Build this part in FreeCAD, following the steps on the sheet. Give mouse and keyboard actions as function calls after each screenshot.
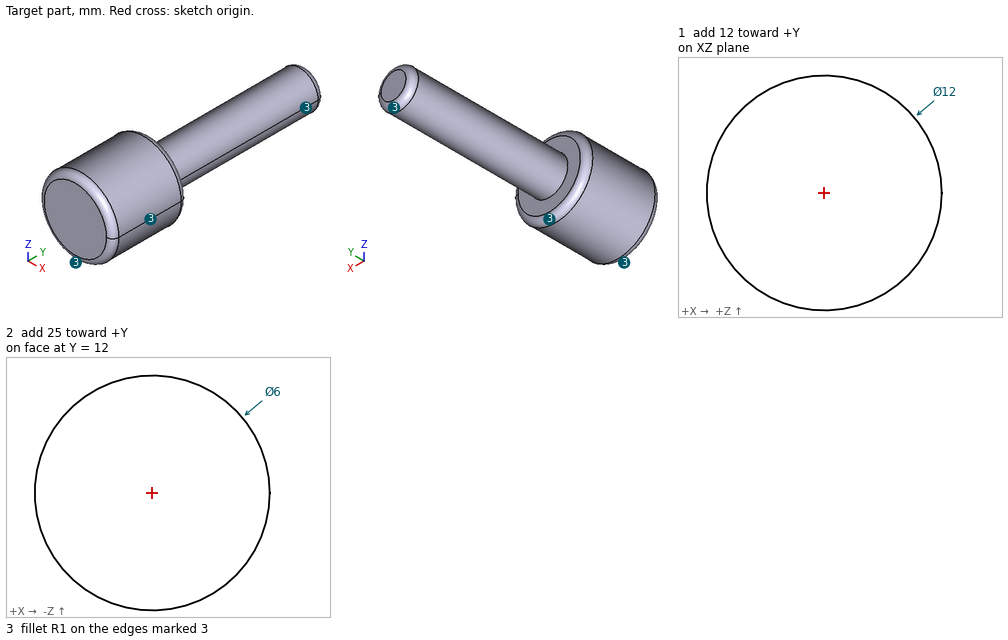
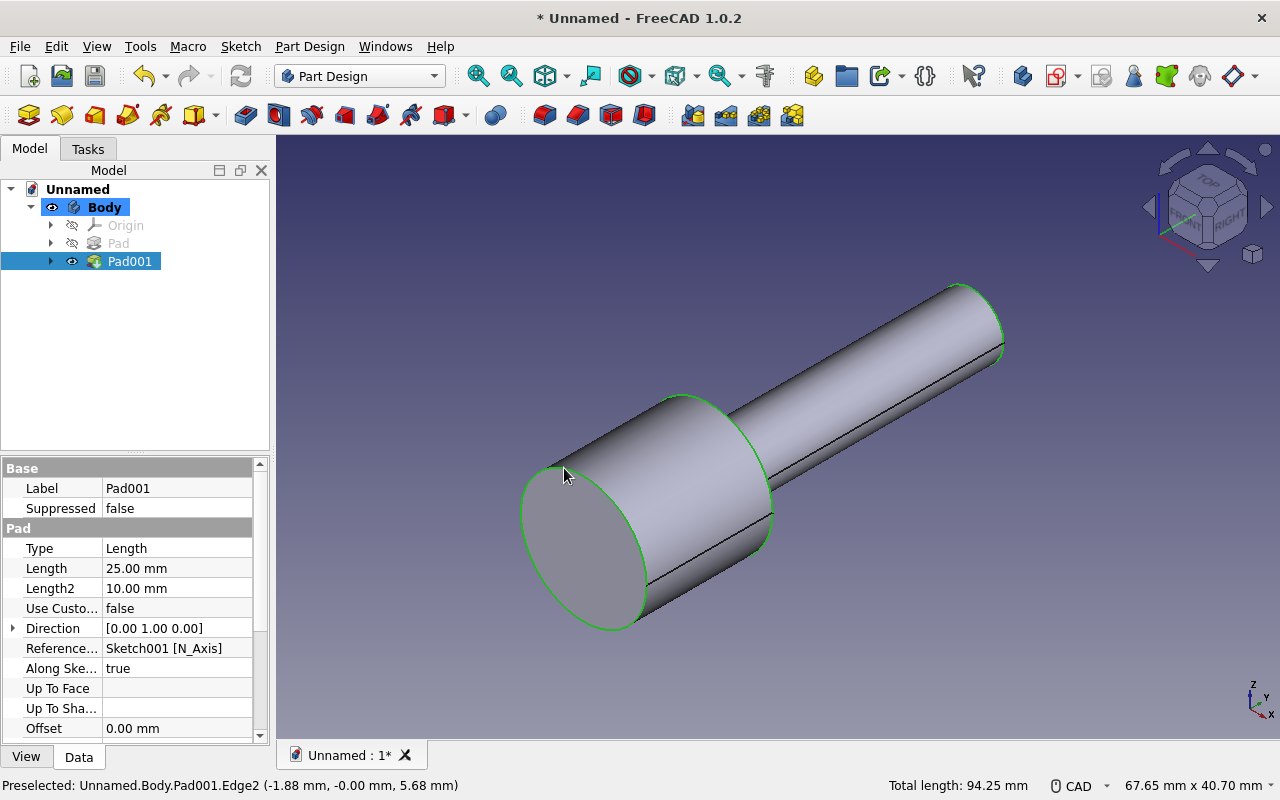
click(545, 116)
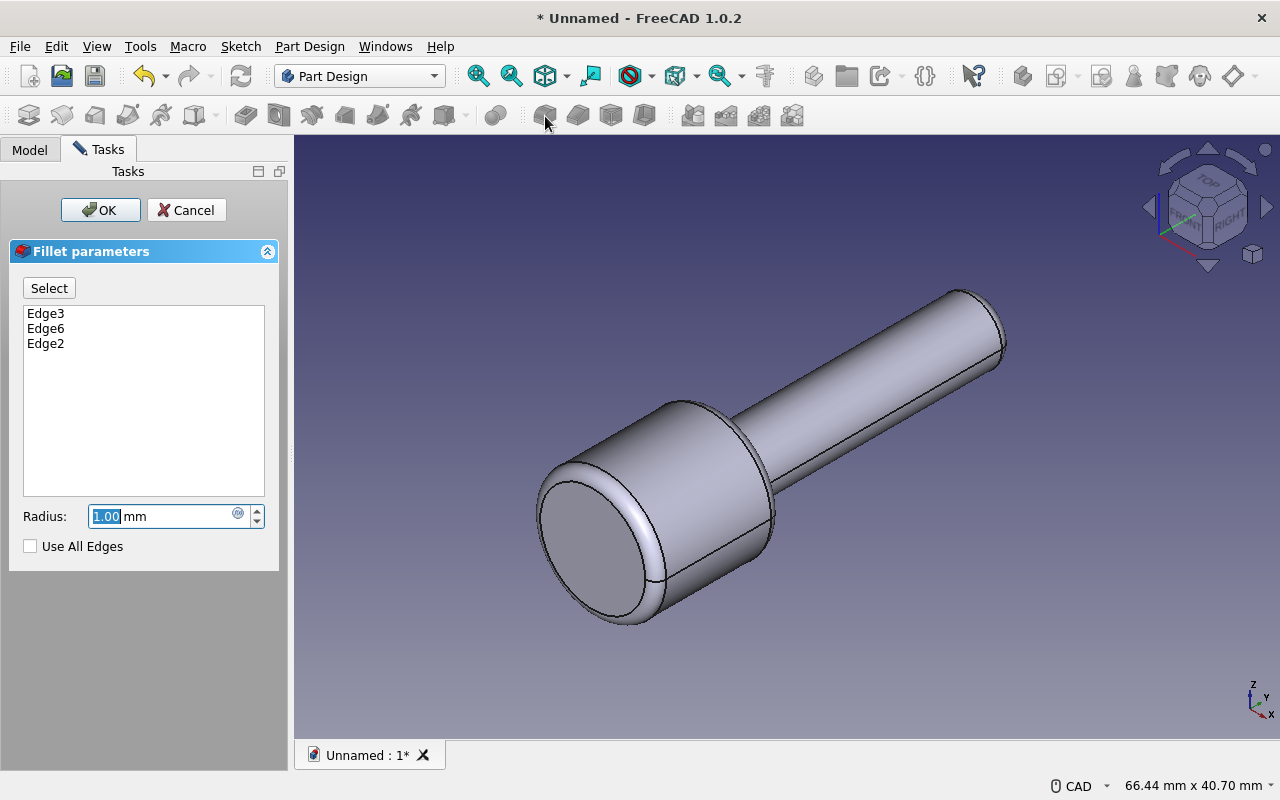
text(1)
key(Tab)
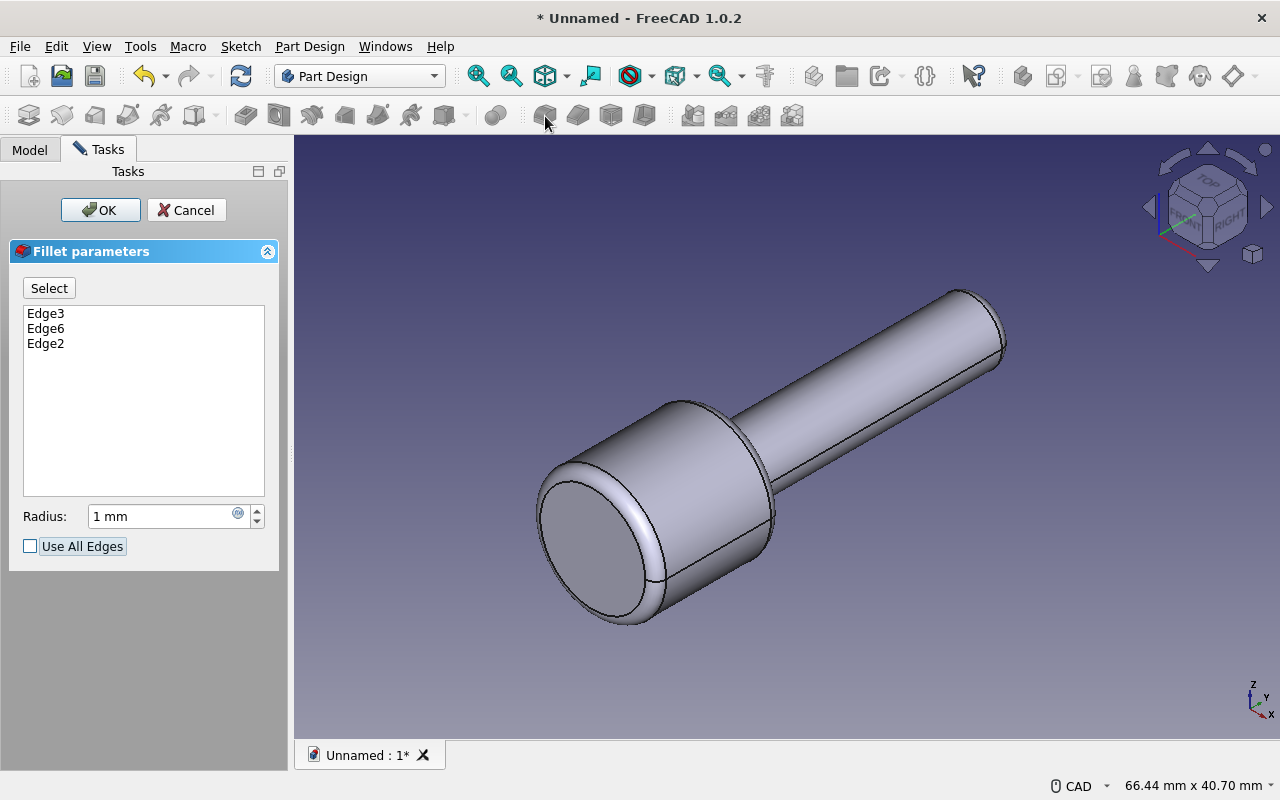
click(101, 210)